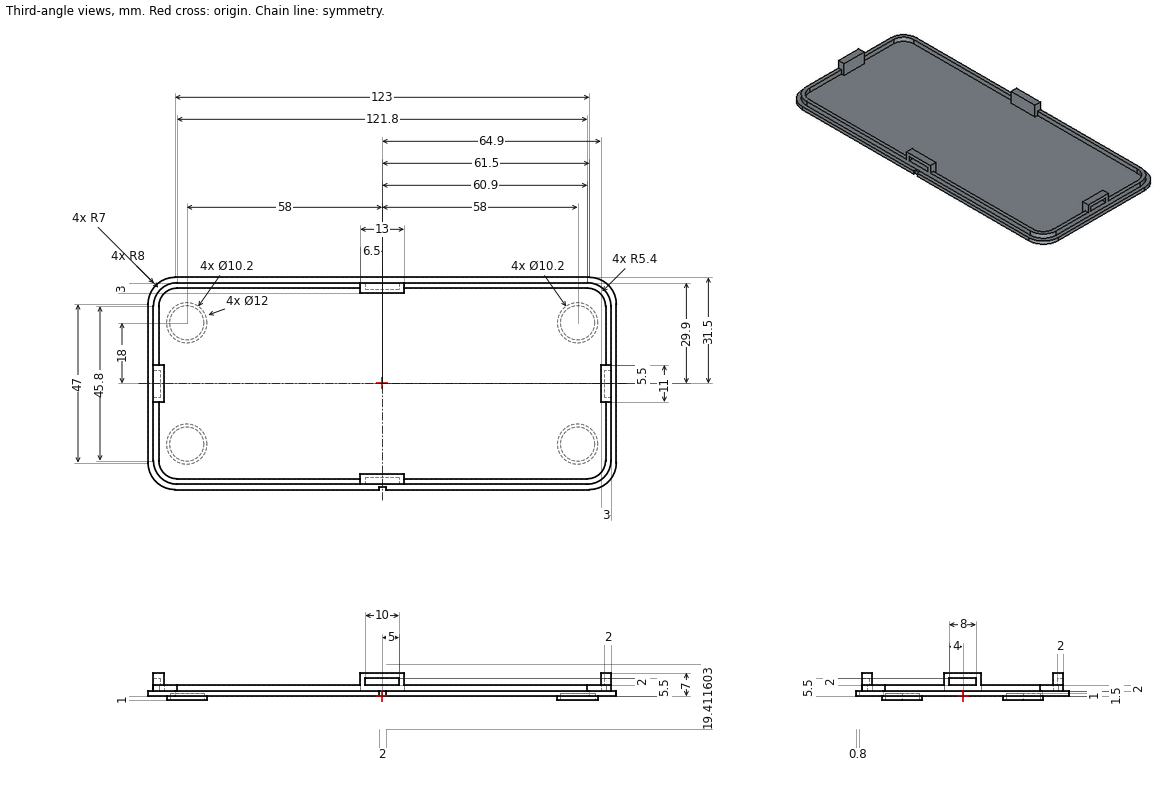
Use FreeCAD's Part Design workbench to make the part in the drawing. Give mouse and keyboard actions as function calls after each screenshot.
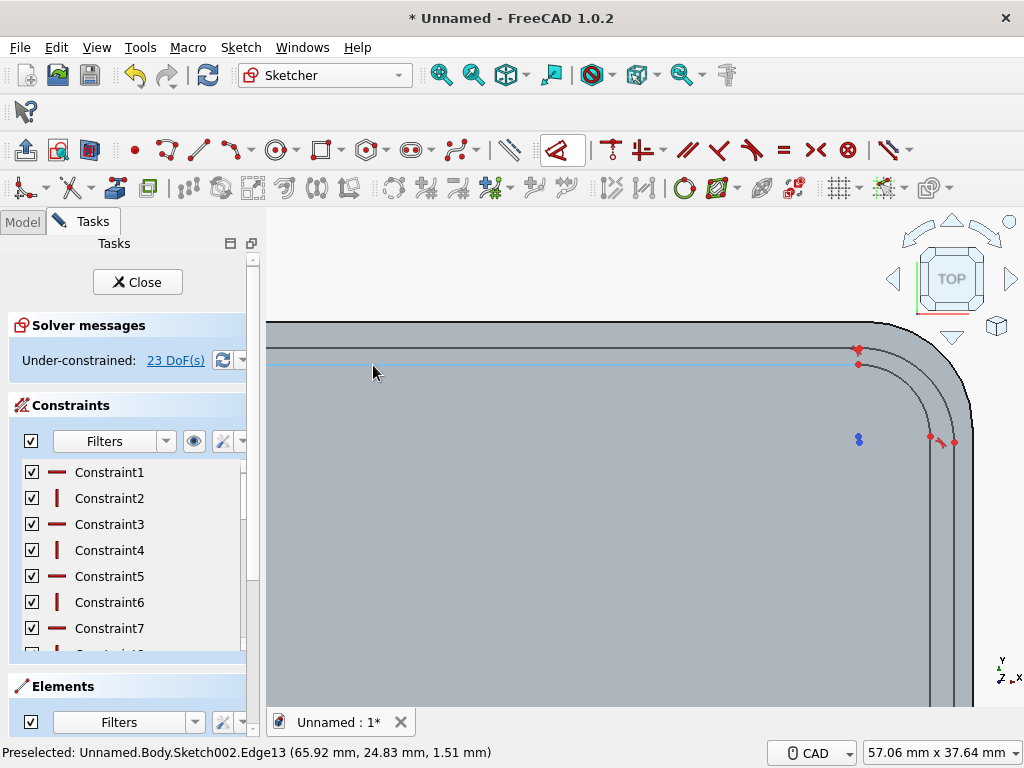
click(373, 365)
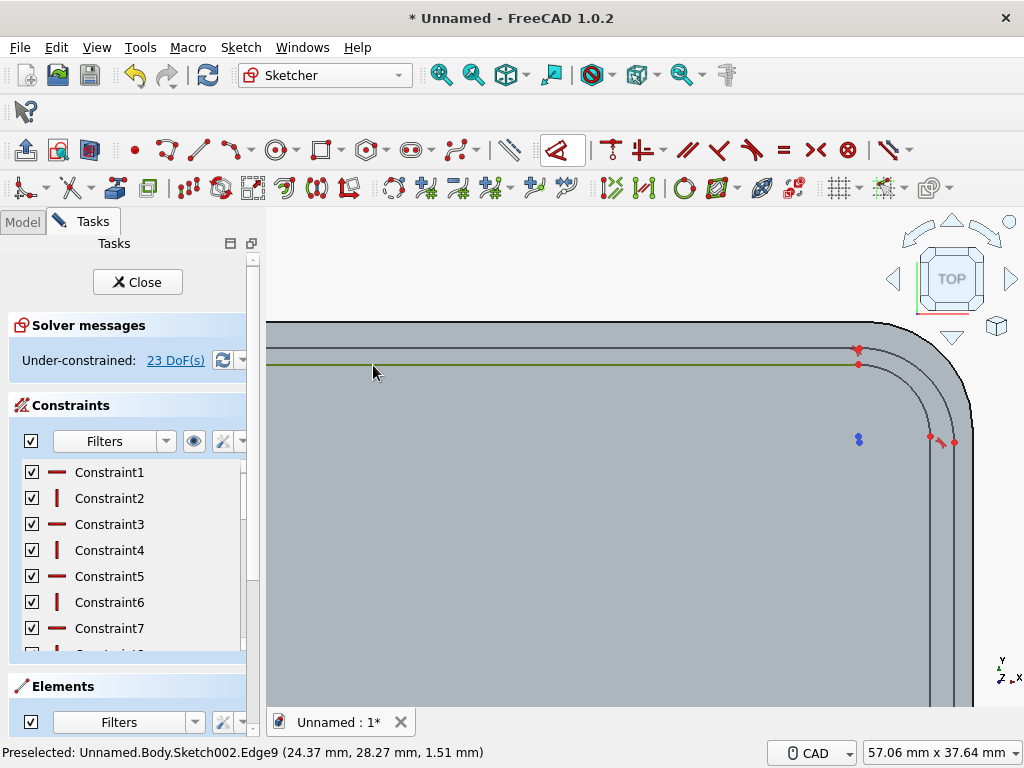
scroll(710, 385, down, 8)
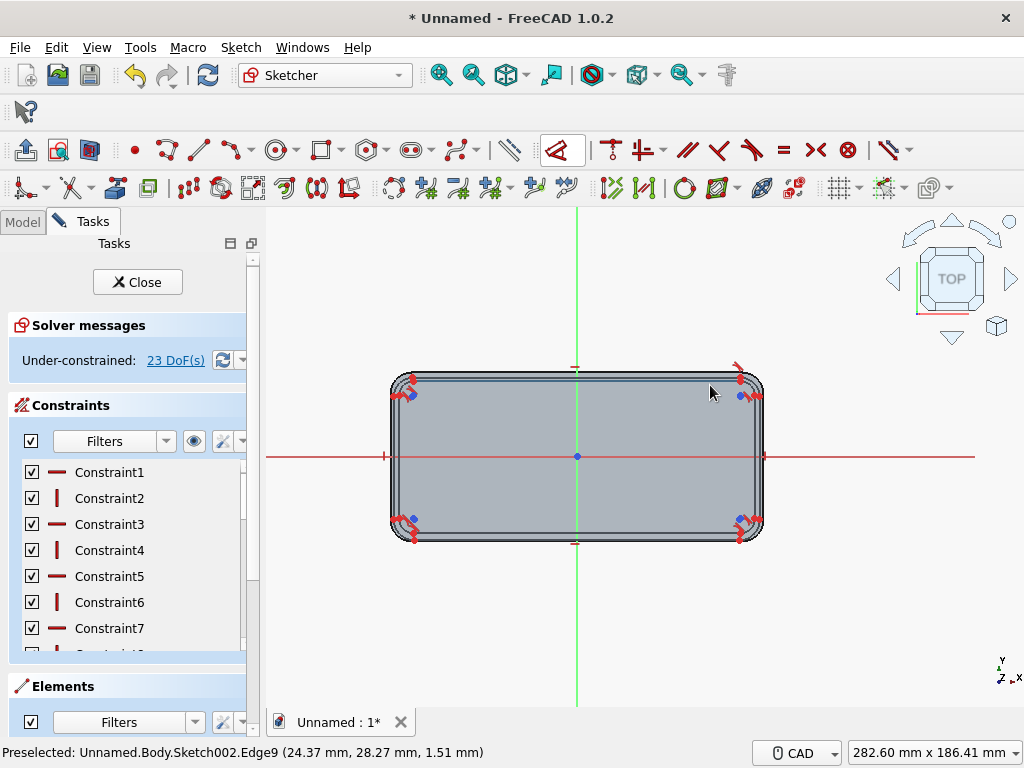
scroll(407, 383, up, 7)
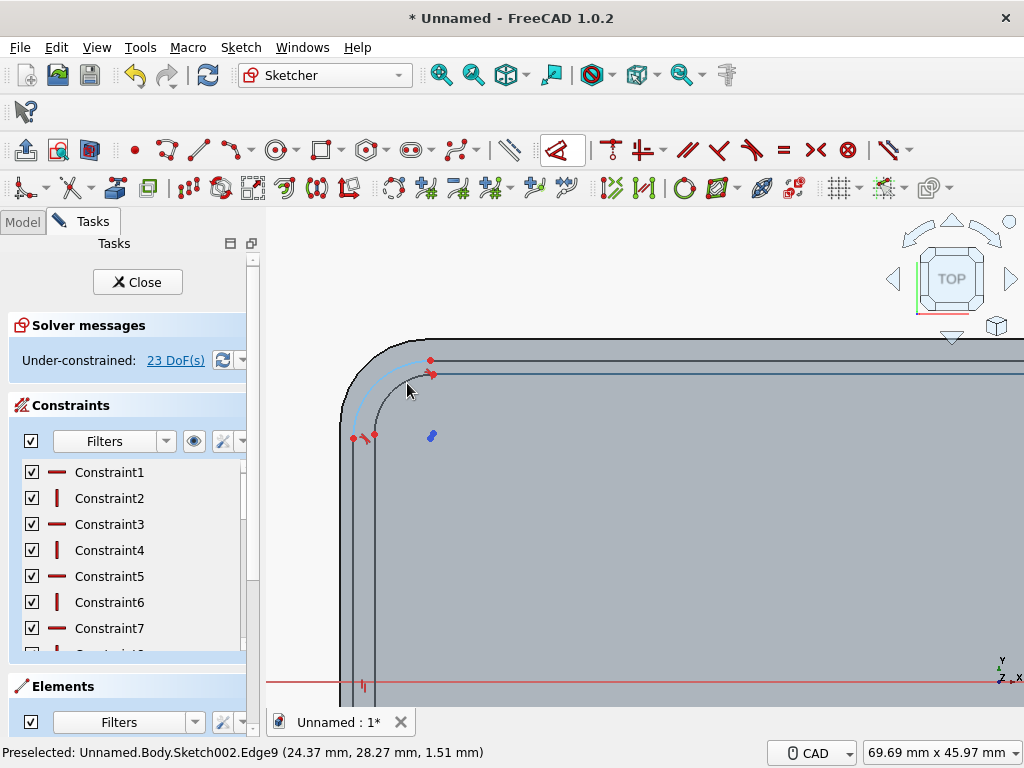
click(407, 381)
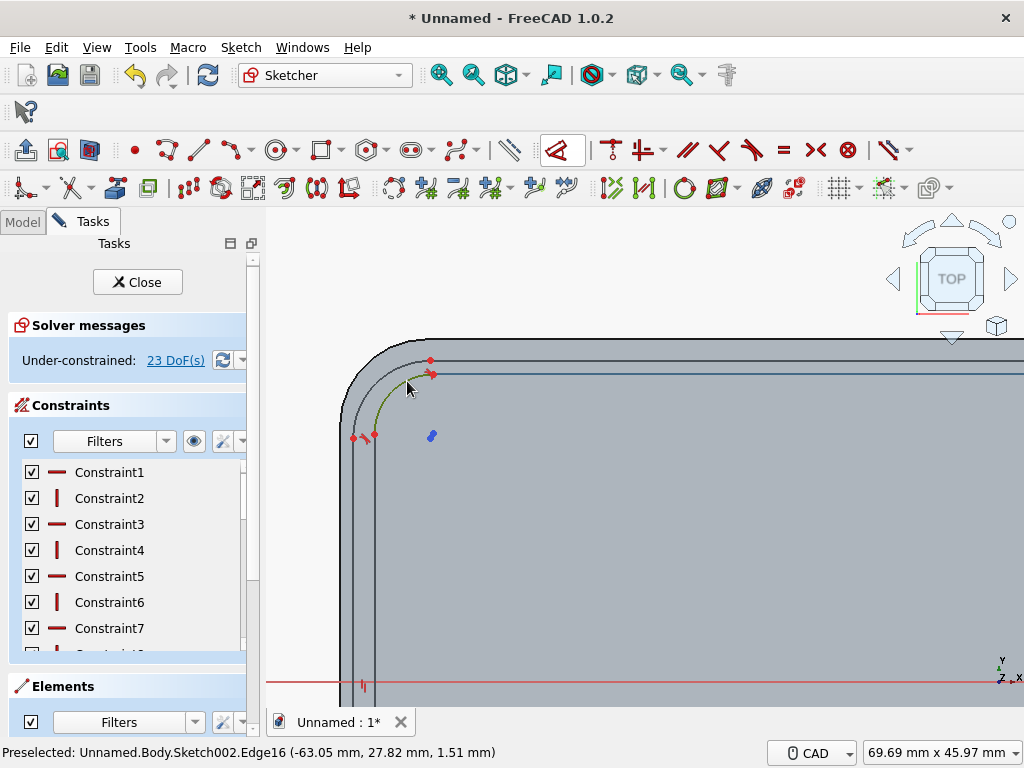
key(t)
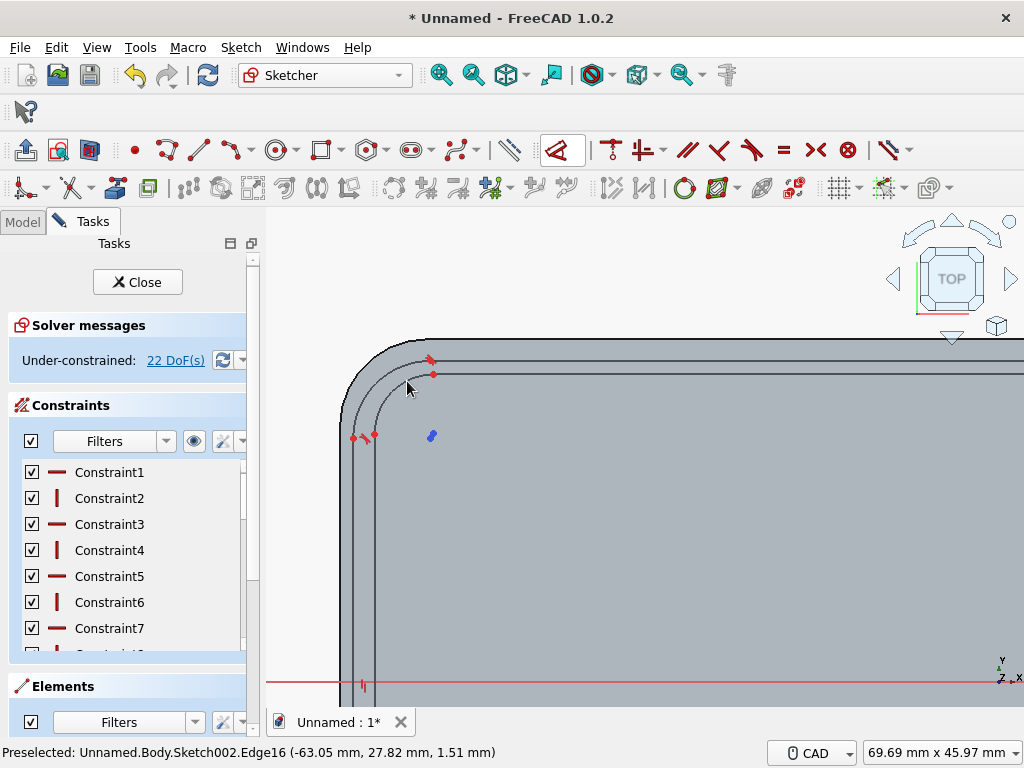
scroll(406, 383, down, 7)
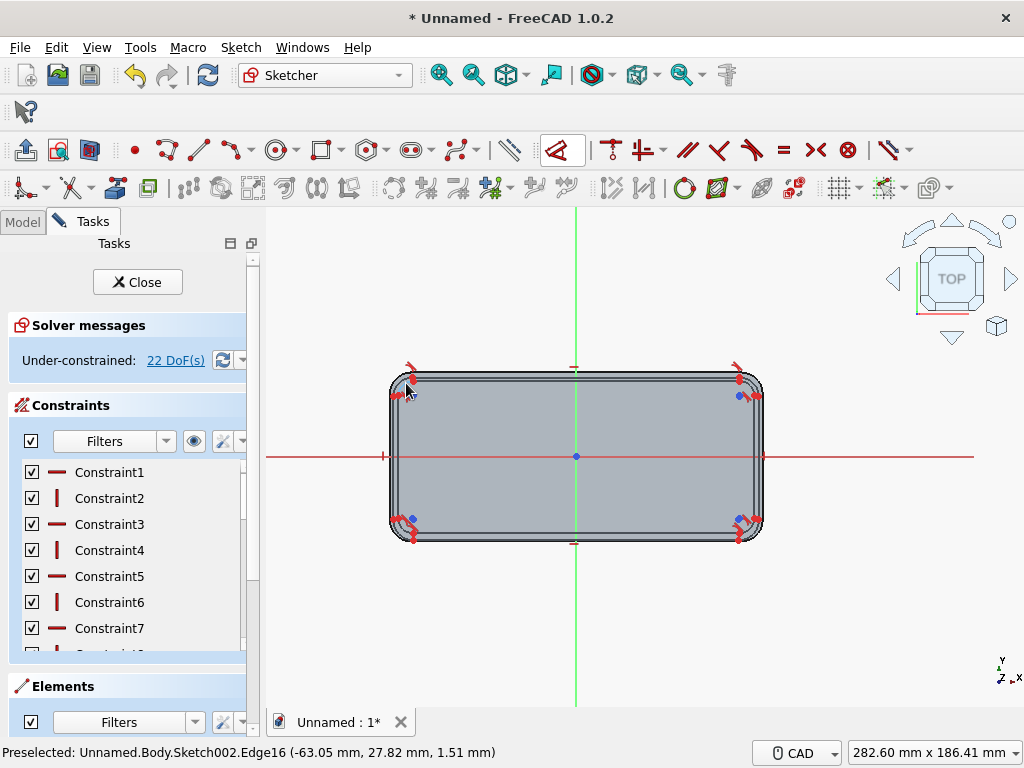
scroll(754, 433, up, 6)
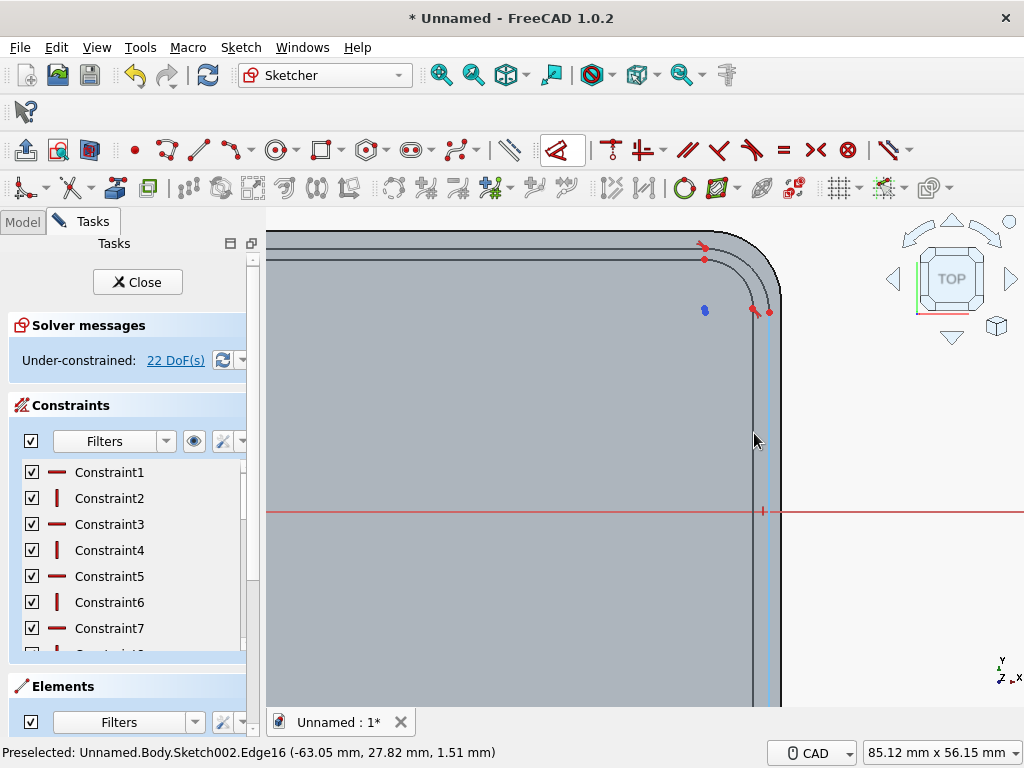
click(753, 431)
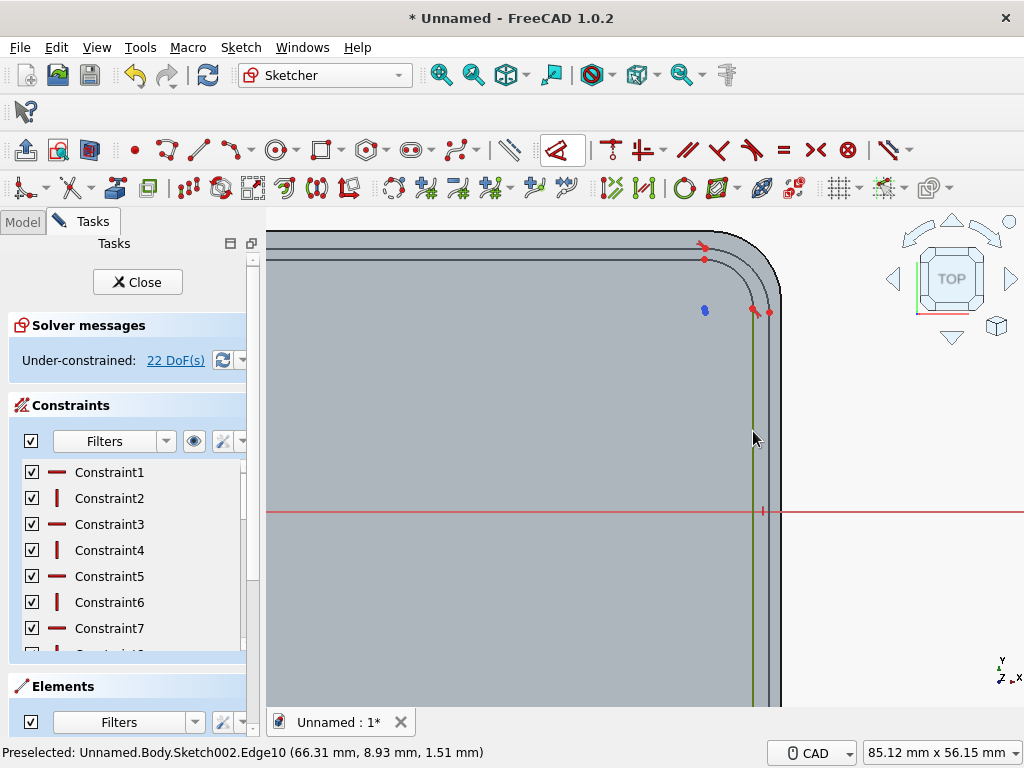
click(748, 286)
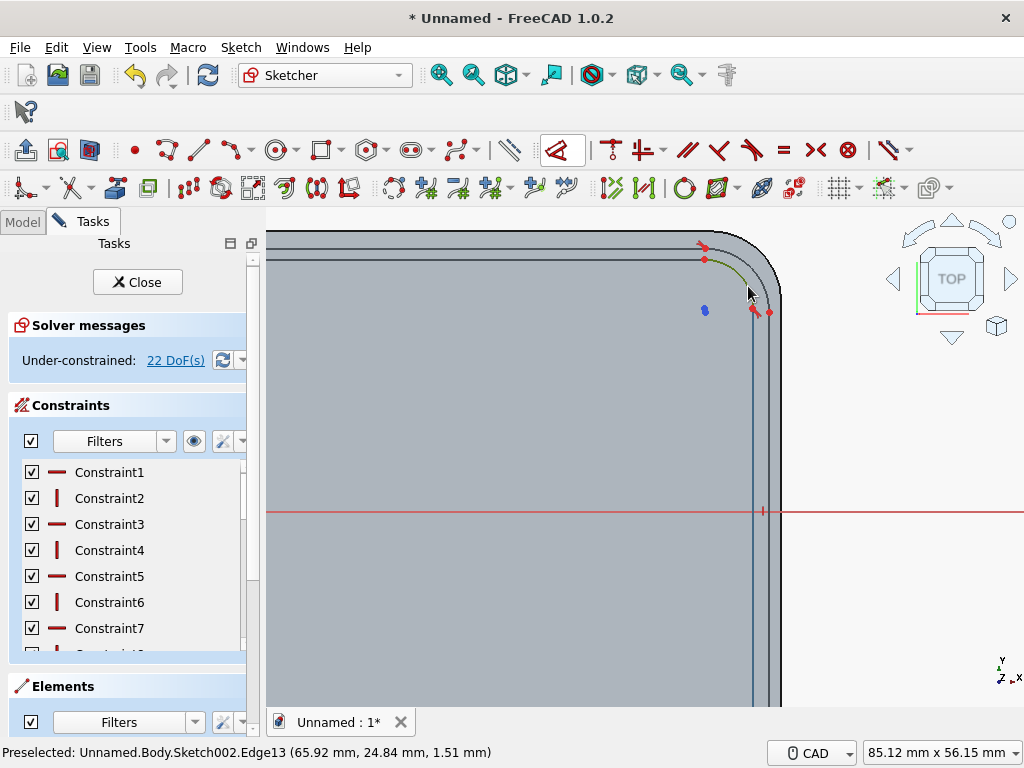
key(t)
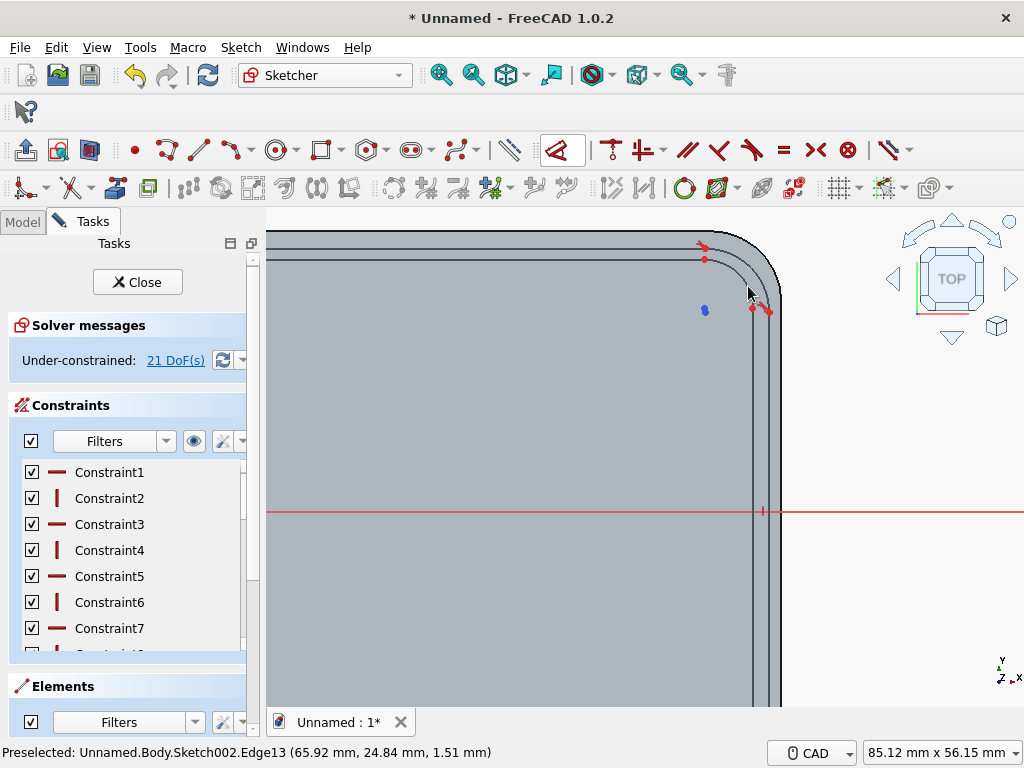
click(753, 431)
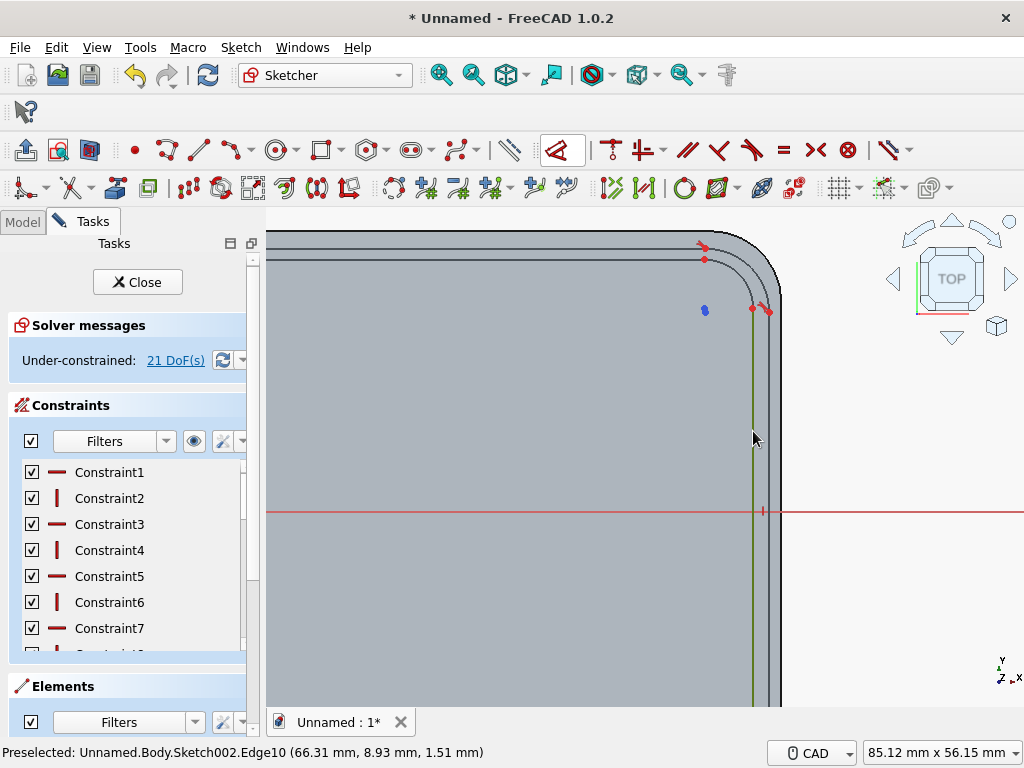
scroll(755, 433, down, 6)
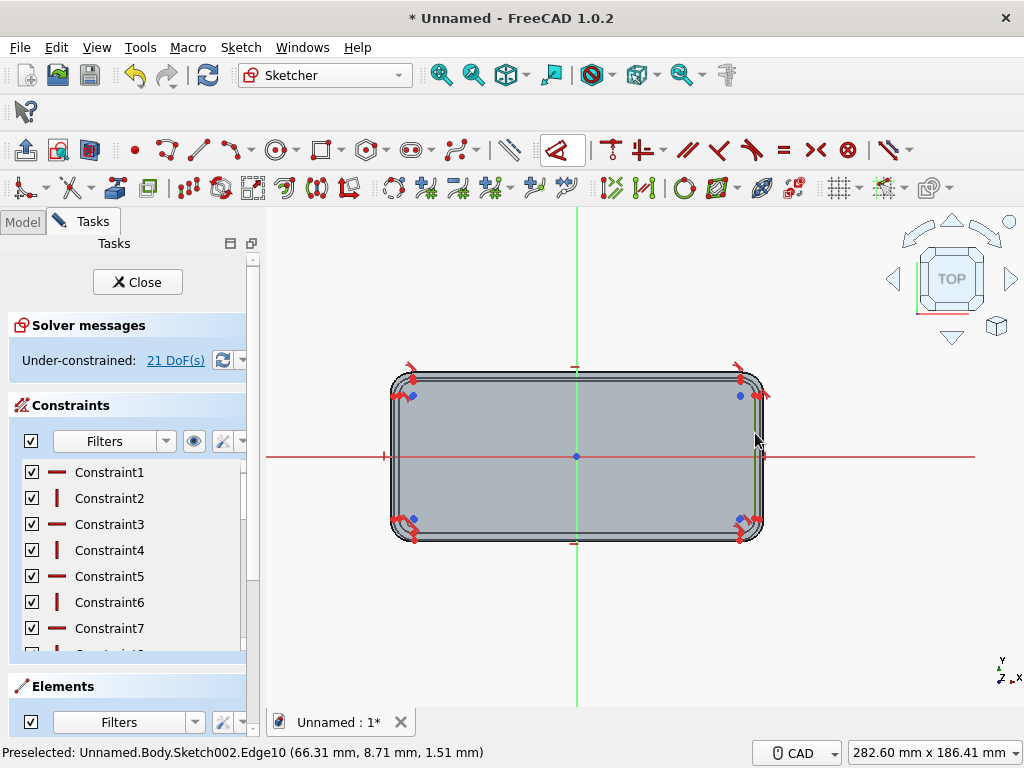
scroll(747, 532, up, 4)